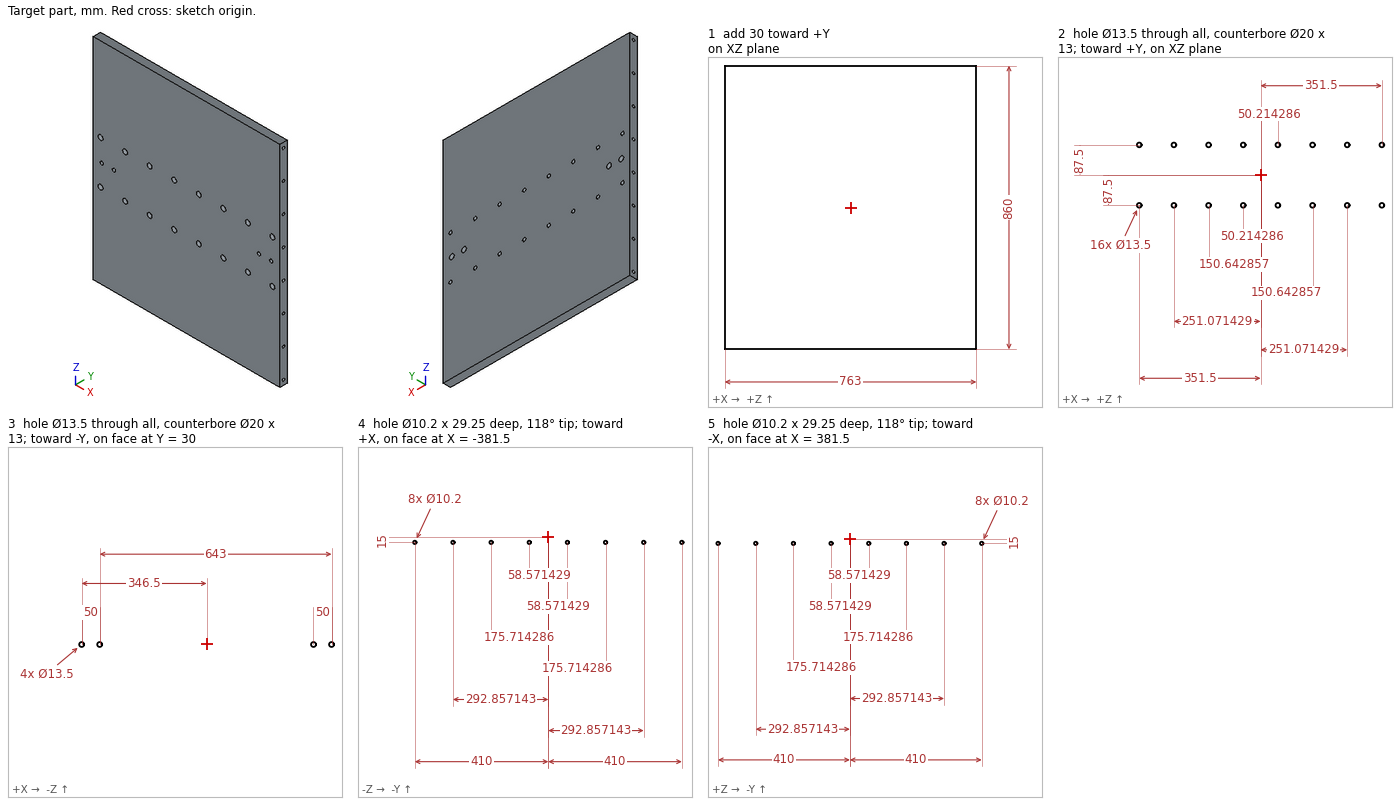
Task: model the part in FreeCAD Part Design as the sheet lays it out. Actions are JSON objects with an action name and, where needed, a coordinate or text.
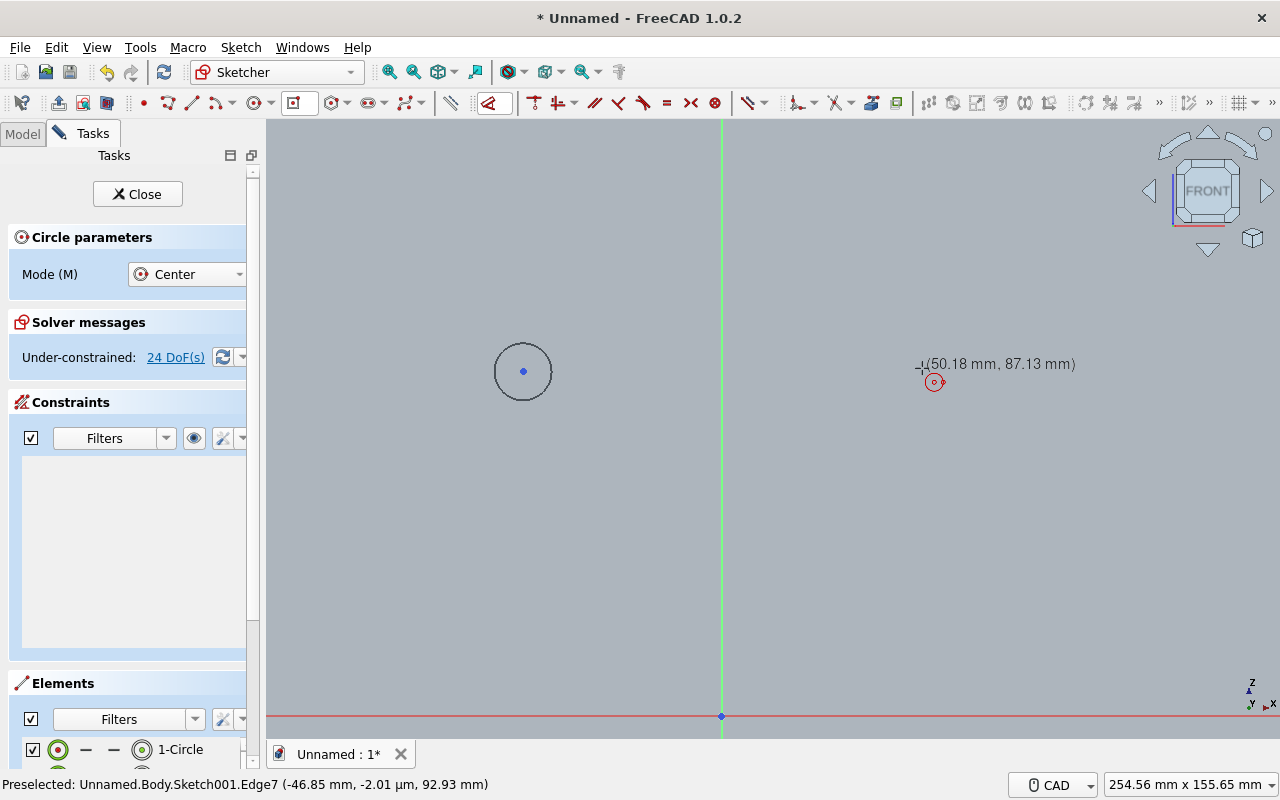
{"action": "scroll", "coordinate": [700, 356], "scroll_direction": "down", "scroll_amount": 8}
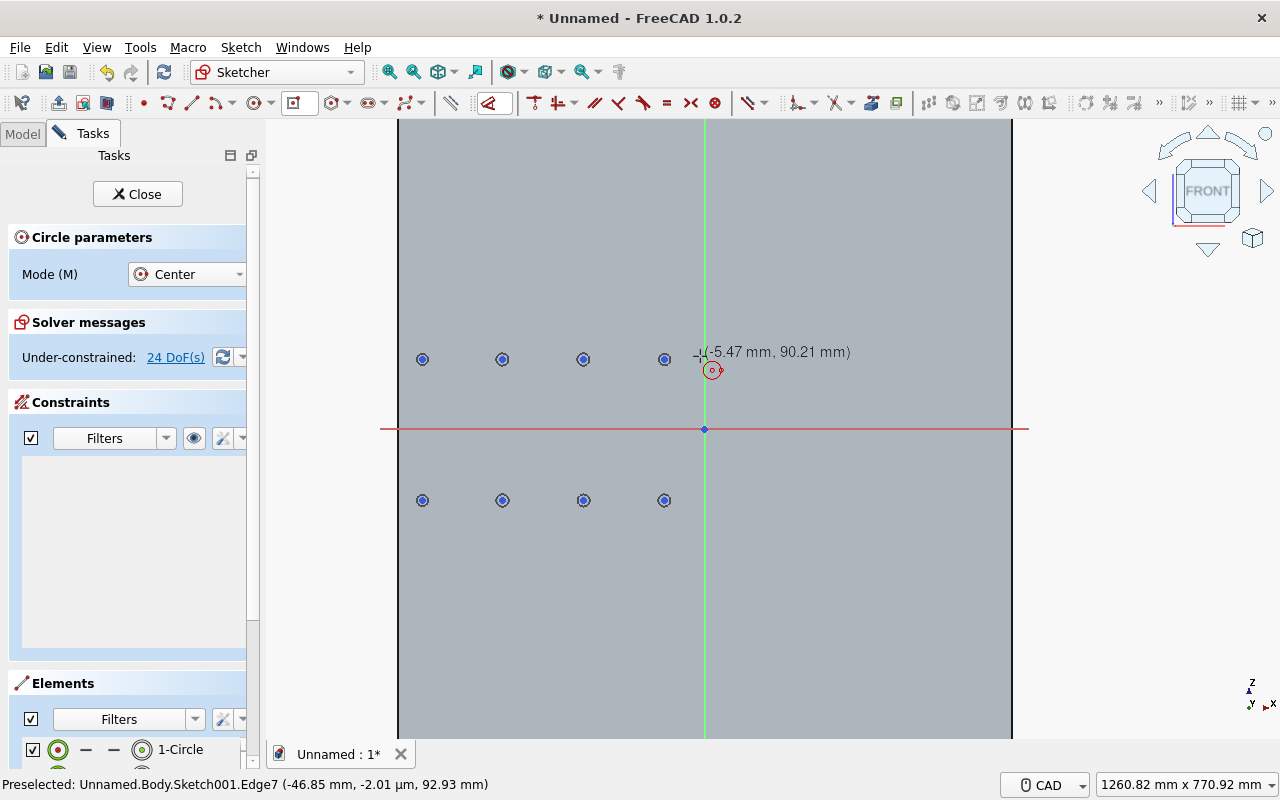
{"action": "left_click", "coordinate": [745, 359]}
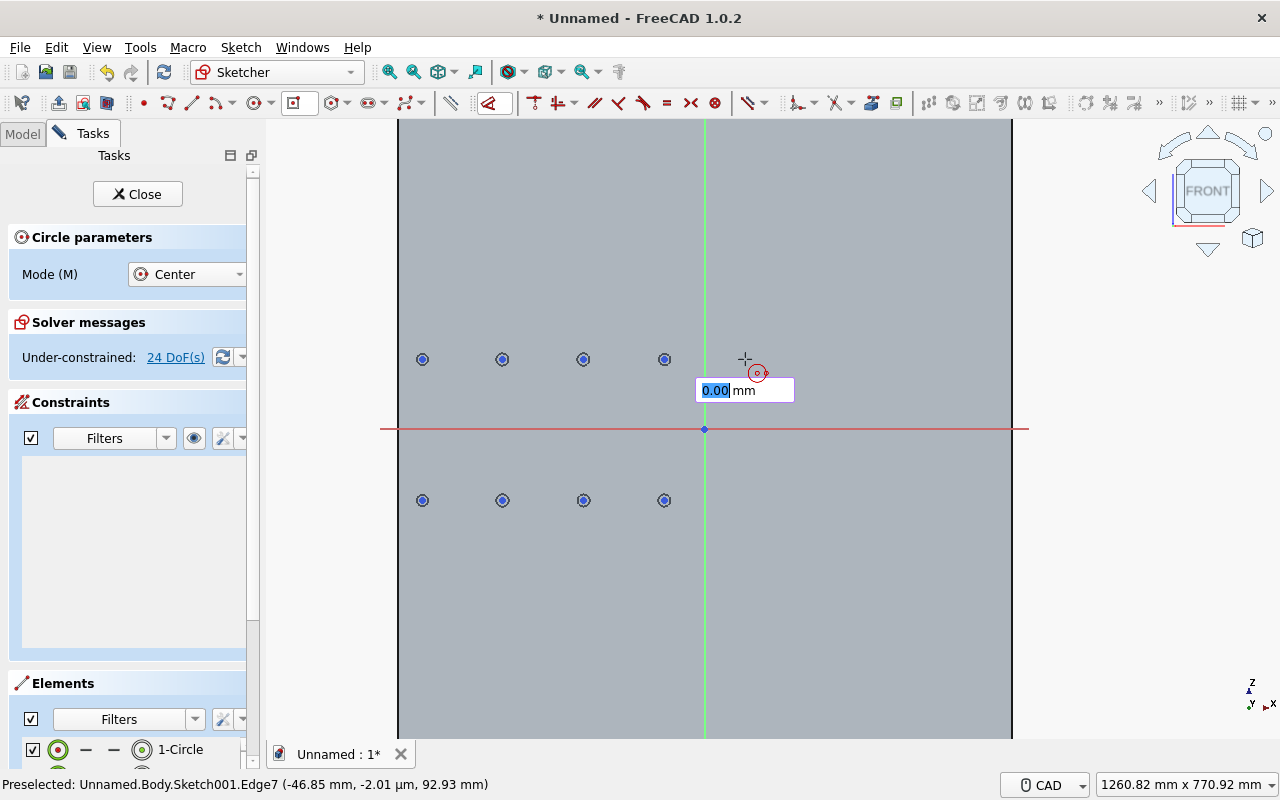
{"action": "scroll", "coordinate": [749, 355], "scroll_direction": "up", "scroll_amount": 6}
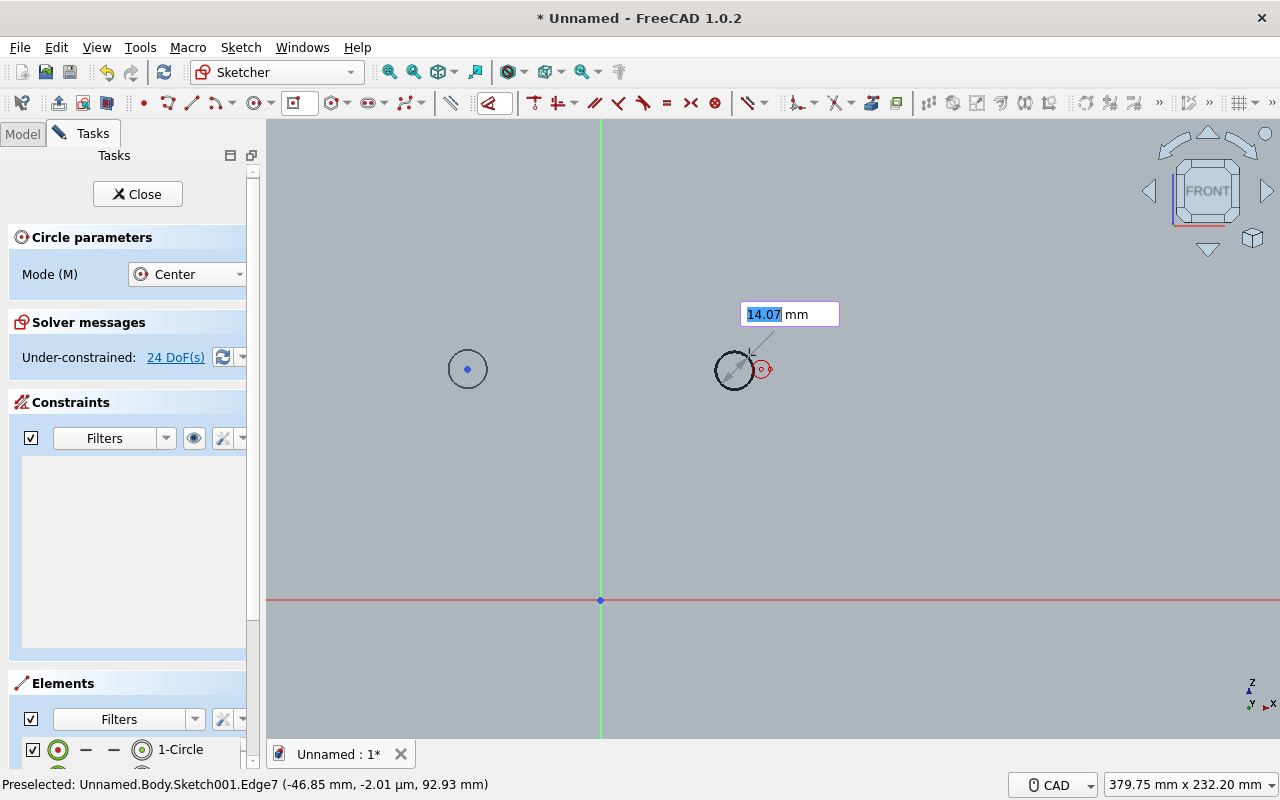
{"action": "left_click", "coordinate": [748, 354]}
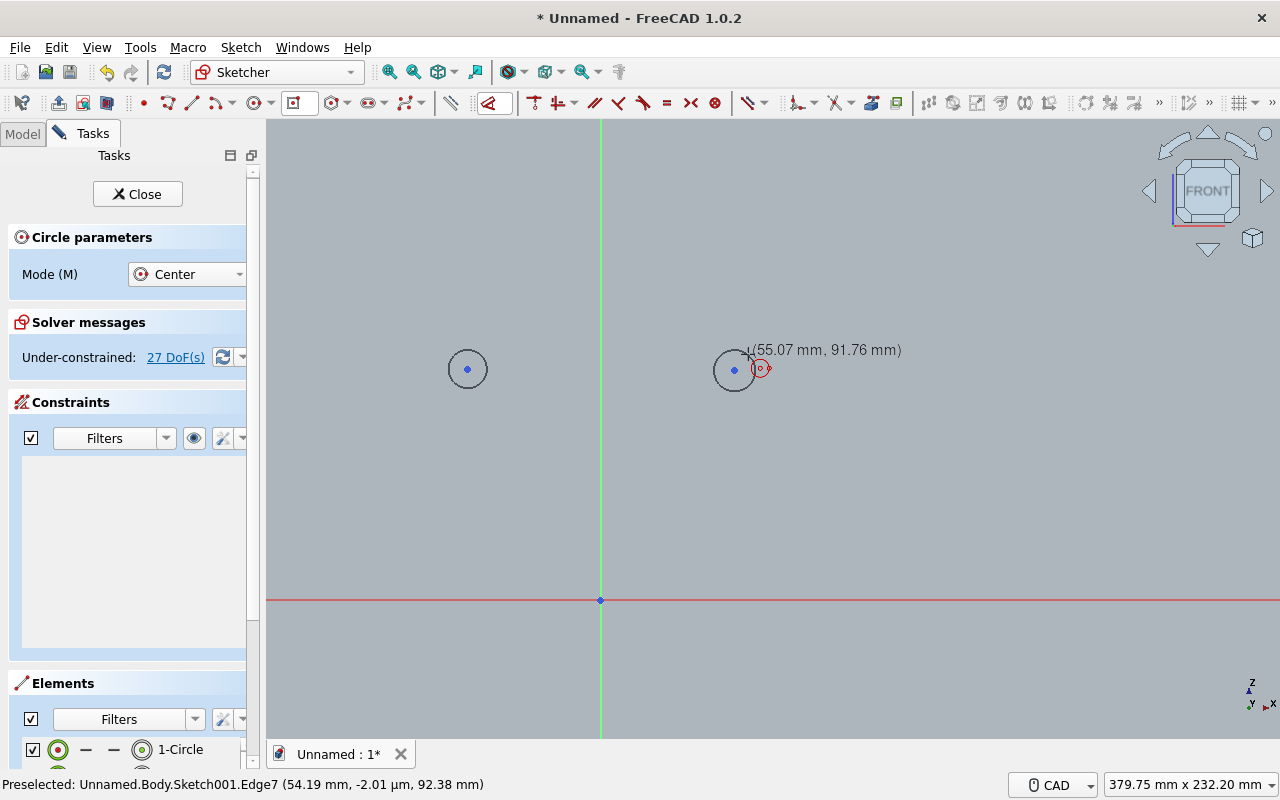
{"action": "scroll", "coordinate": [749, 355], "scroll_direction": "down", "scroll_amount": 6}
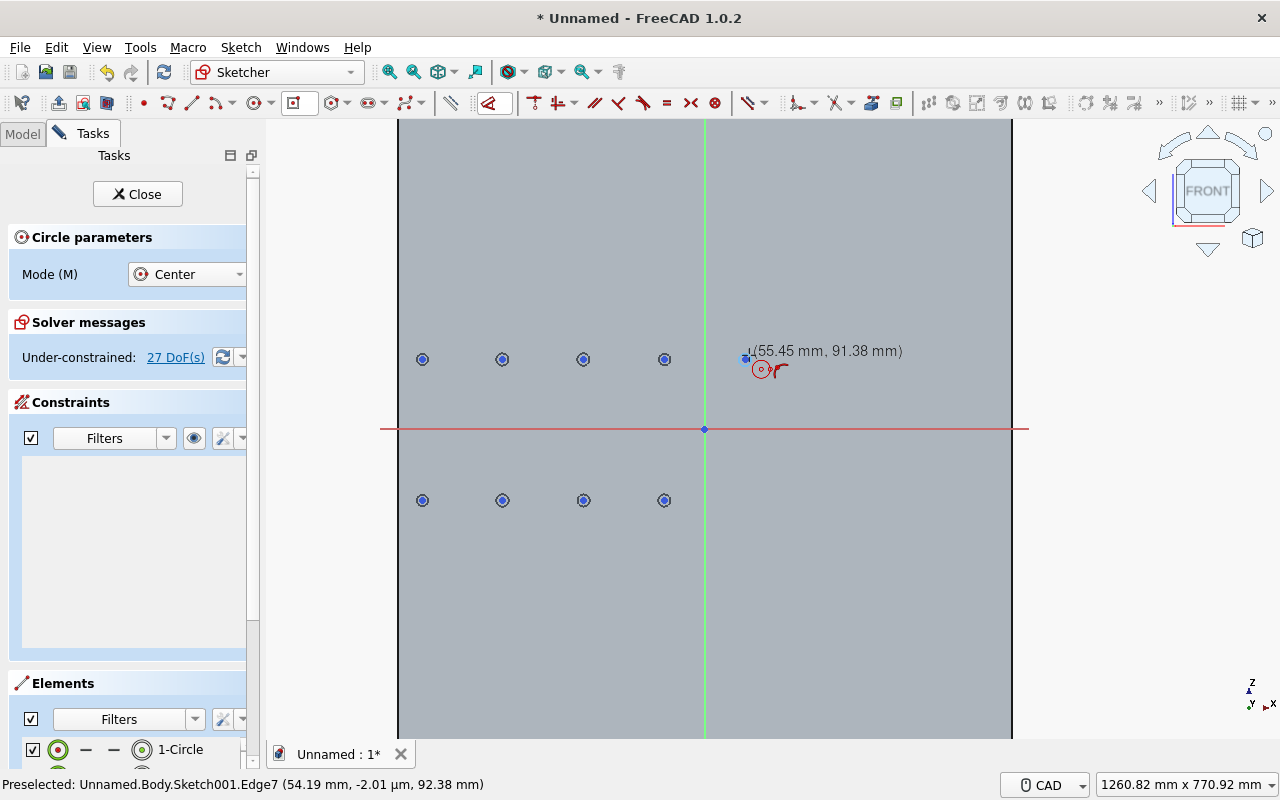
{"action": "scroll", "coordinate": [745, 499], "scroll_direction": "up", "scroll_amount": 8}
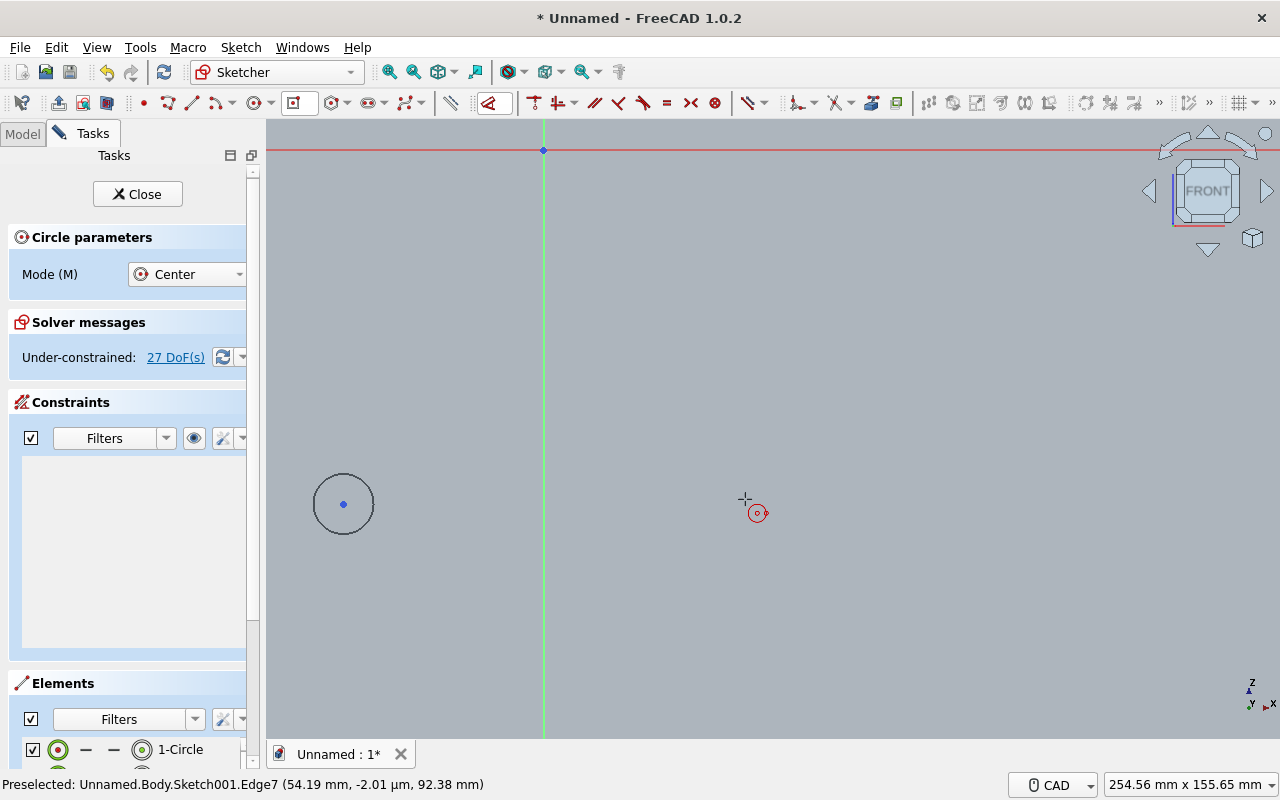
{"action": "scroll", "coordinate": [745, 500], "scroll_direction": "down", "scroll_amount": 8}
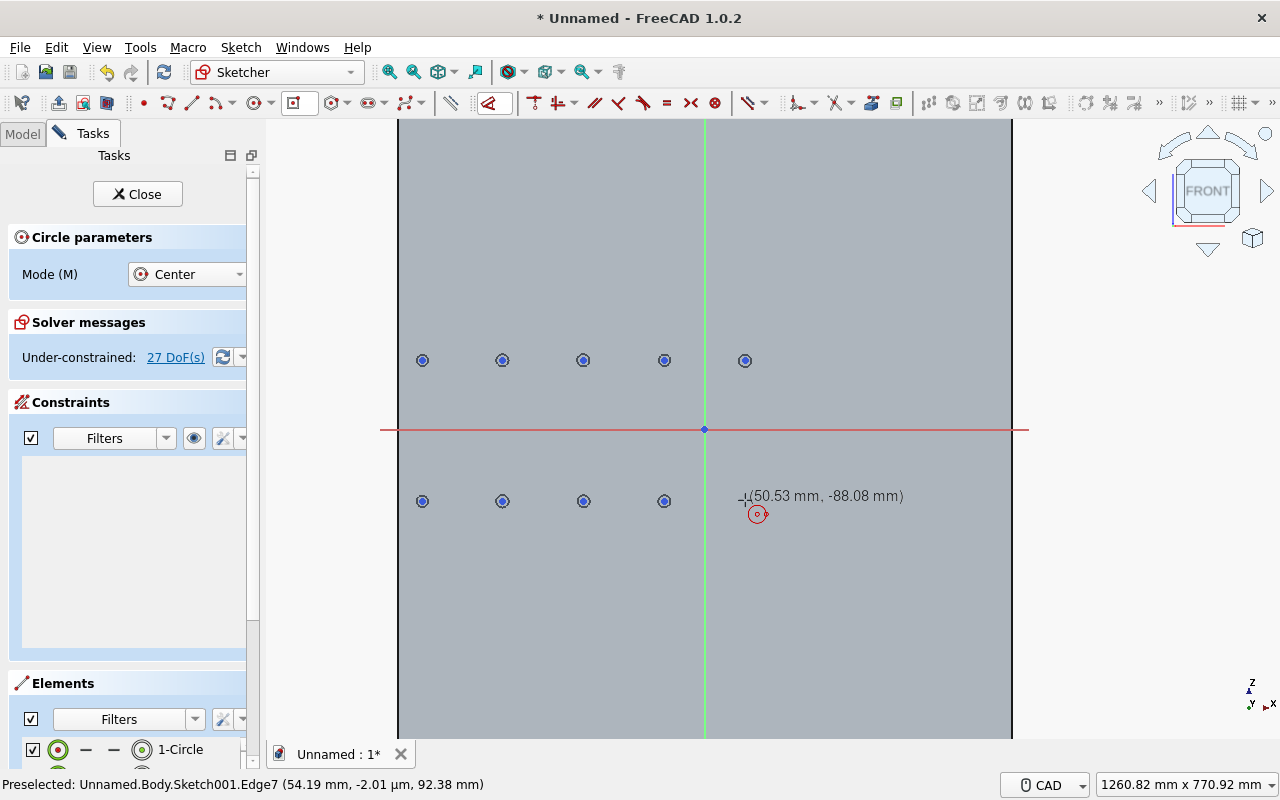
{"action": "left_click", "coordinate": [745, 500]}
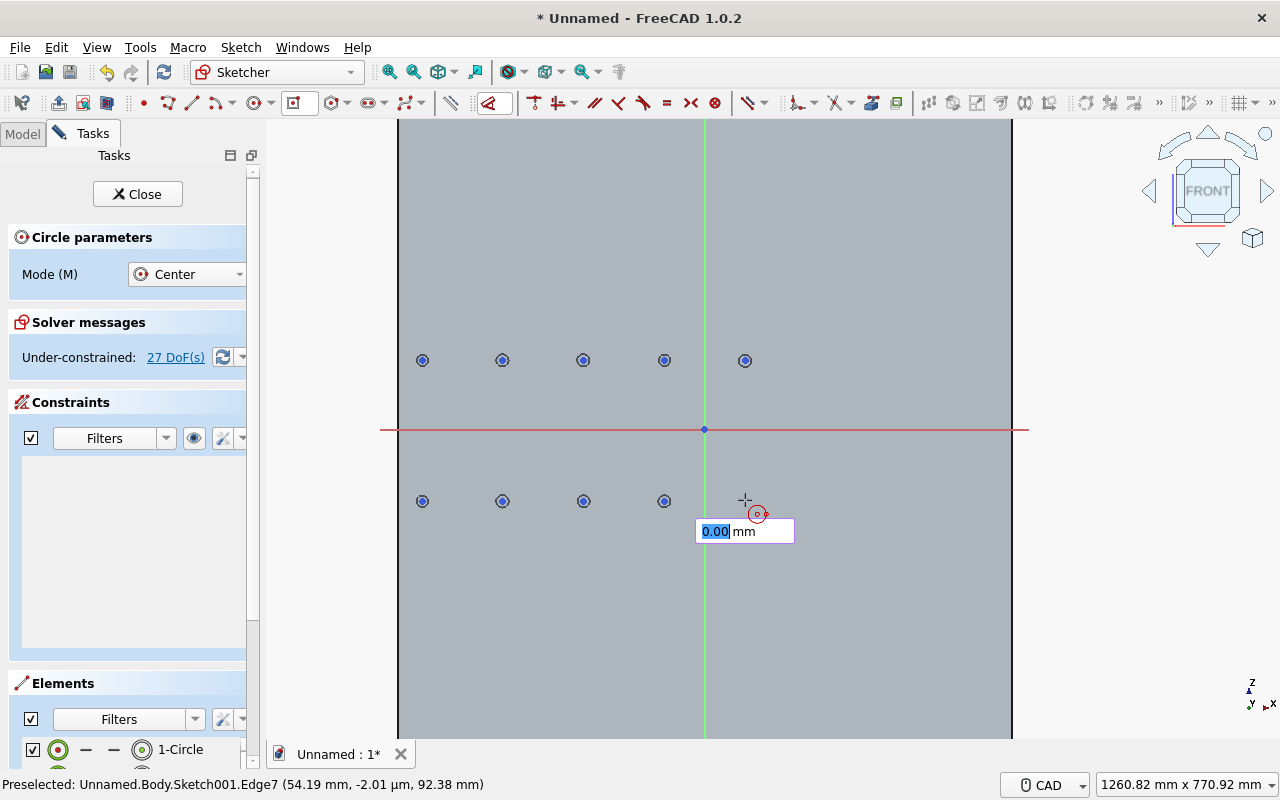
{"action": "scroll", "coordinate": [749, 496], "scroll_direction": "up", "scroll_amount": 6}